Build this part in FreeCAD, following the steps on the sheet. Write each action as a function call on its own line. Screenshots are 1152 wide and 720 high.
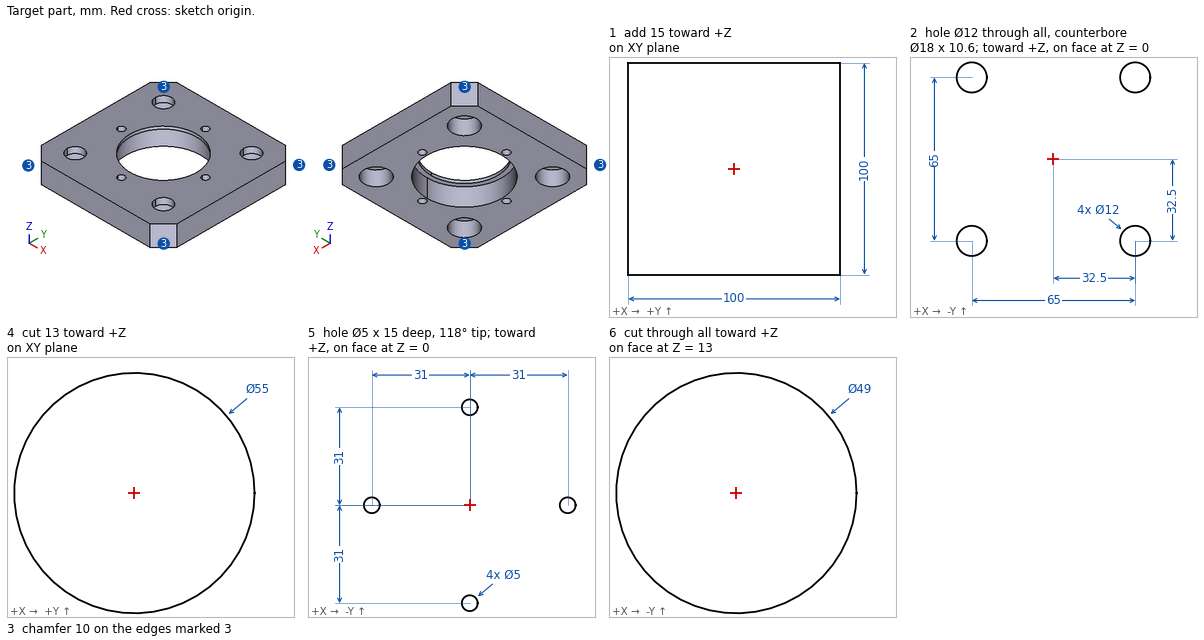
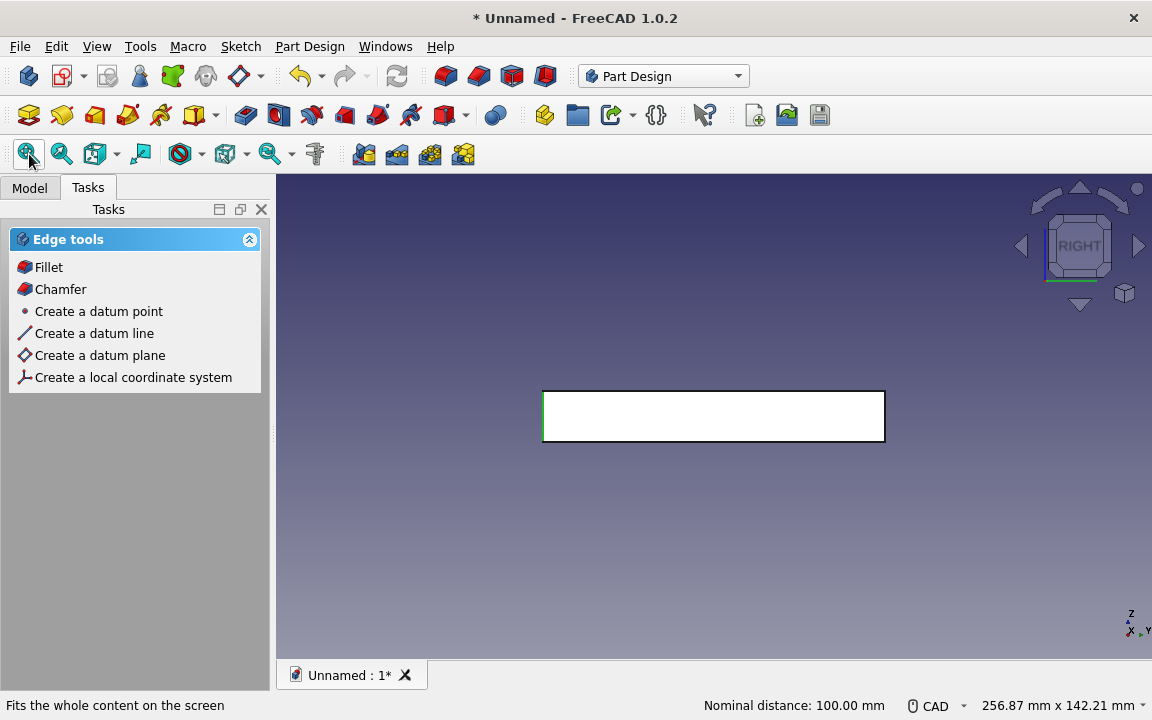
click(885, 415, ctrl)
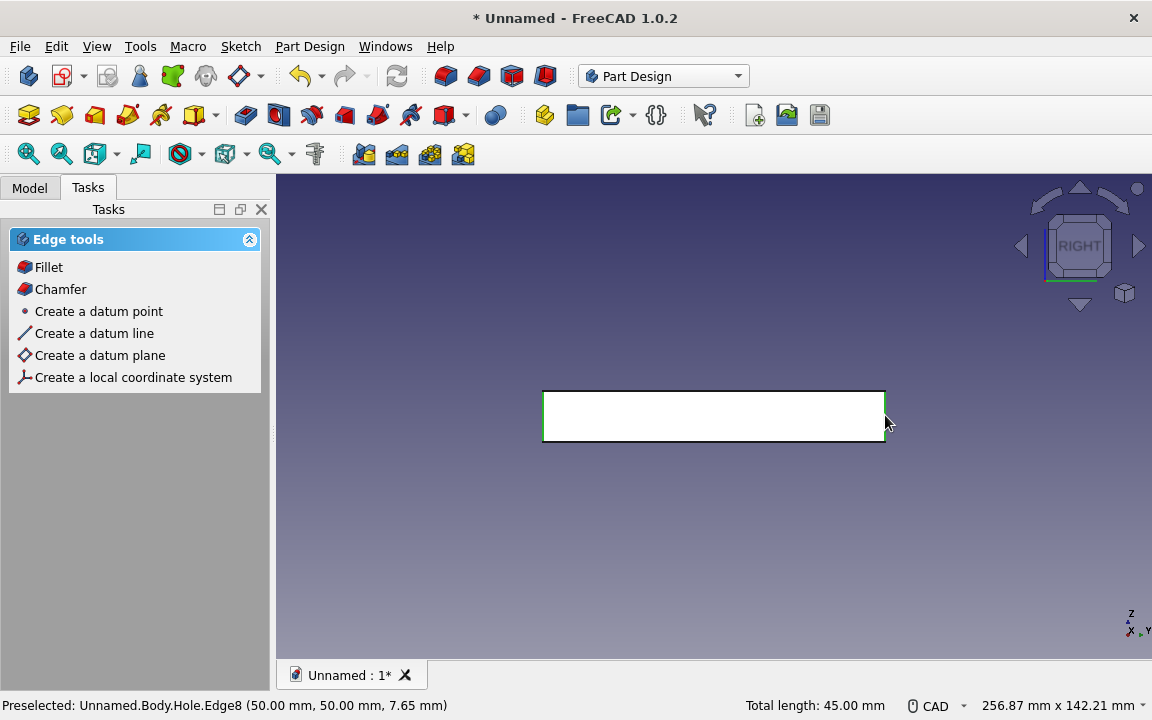
key(5)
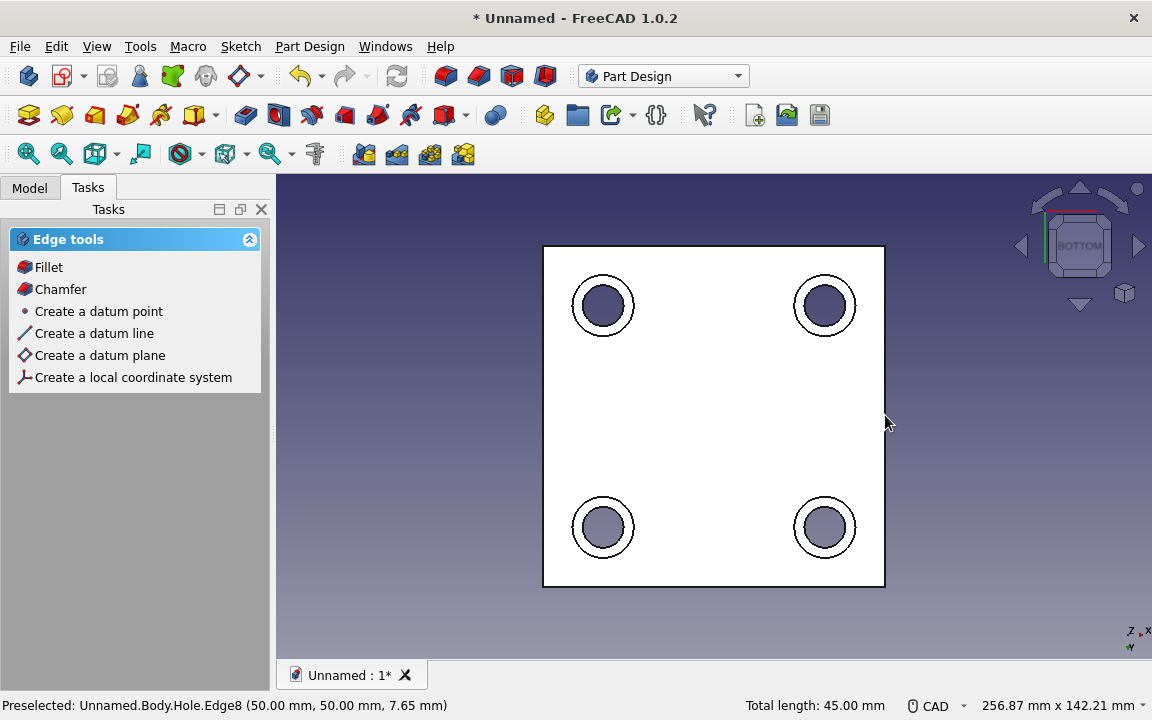
key(4)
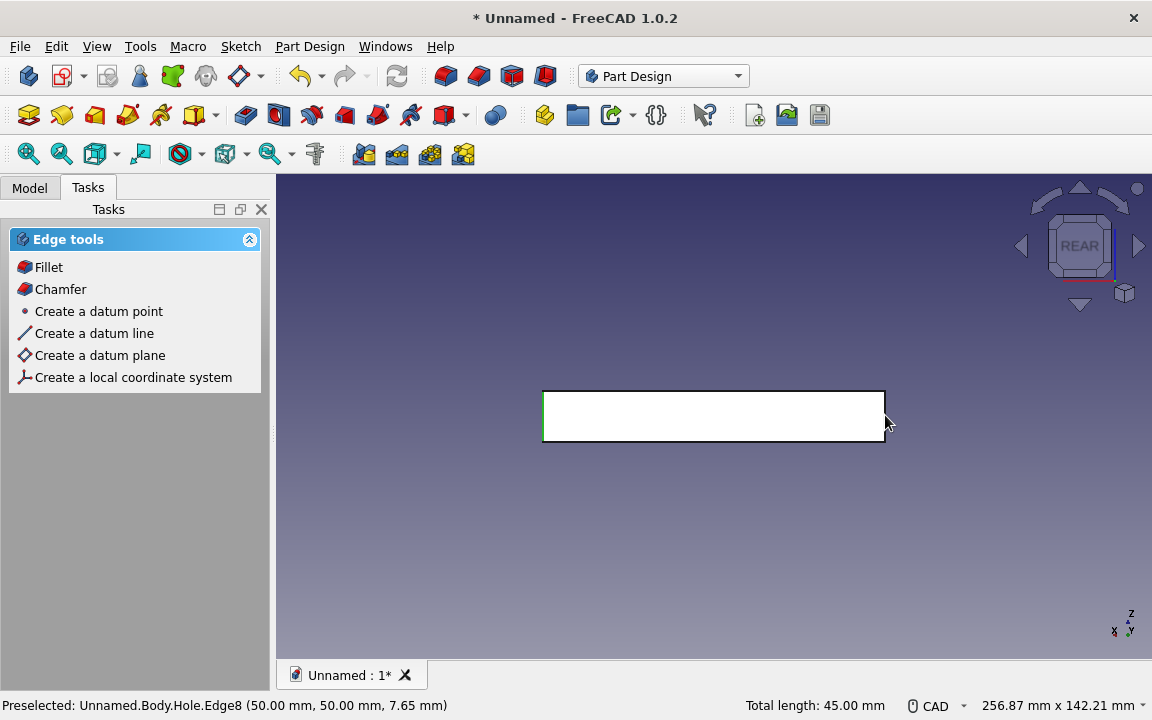
click(29, 154)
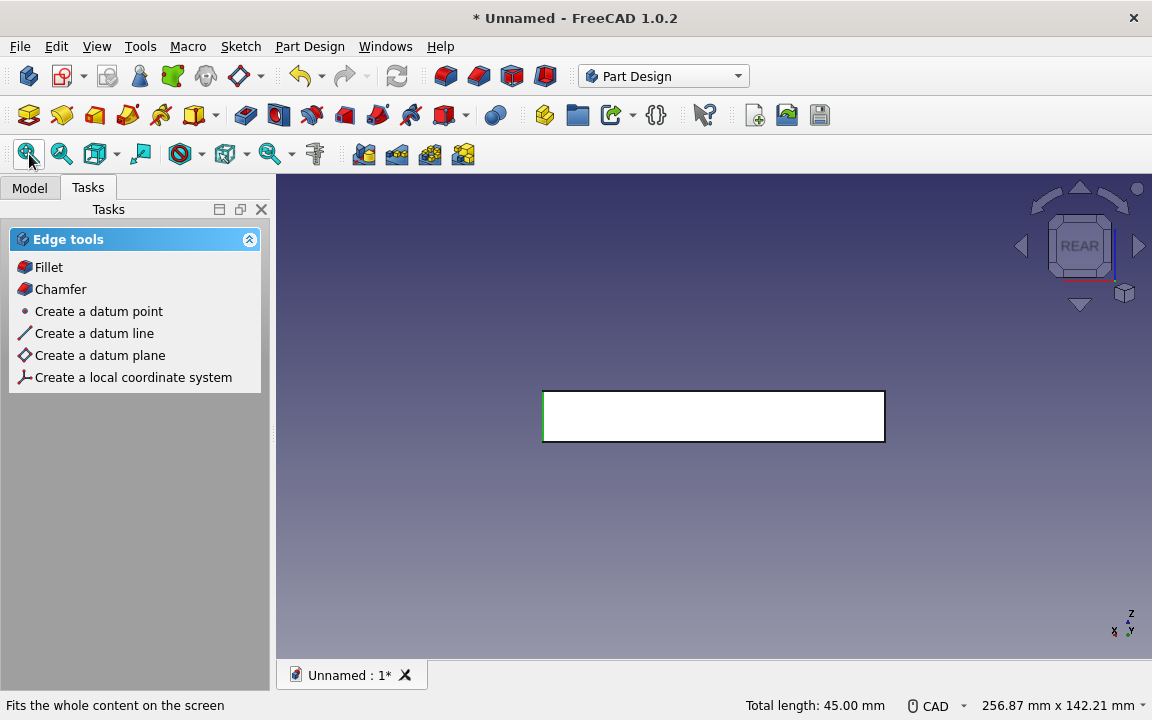
click(885, 416, ctrl)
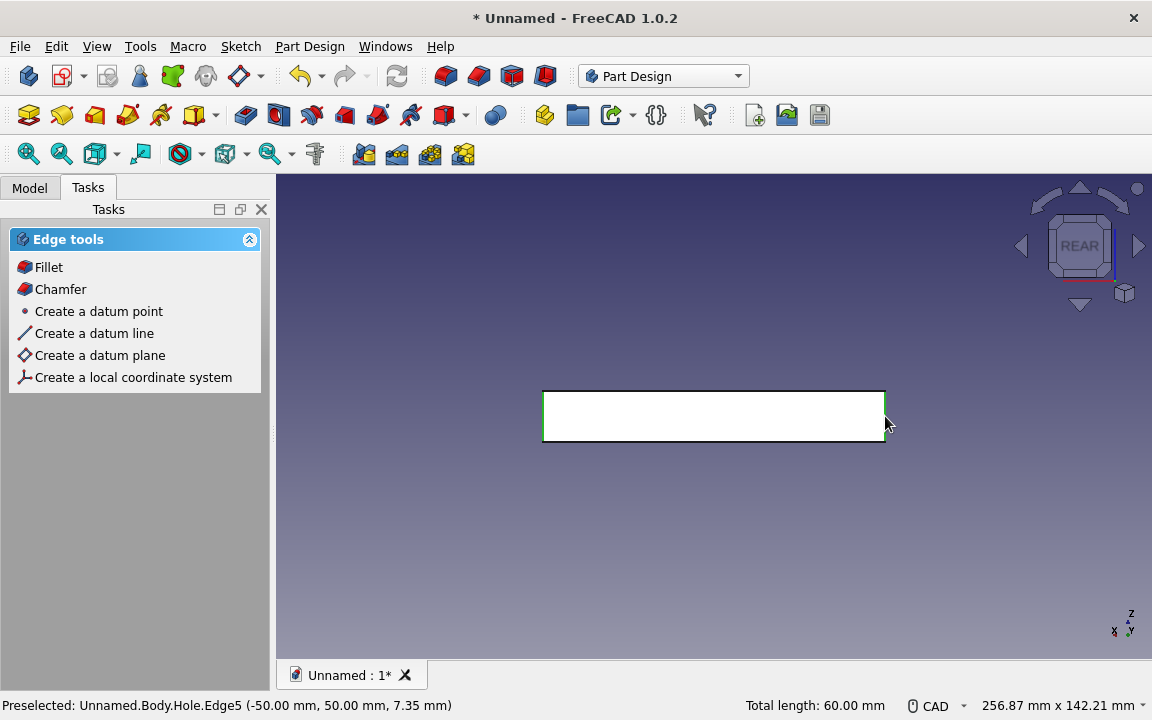
click(479, 76)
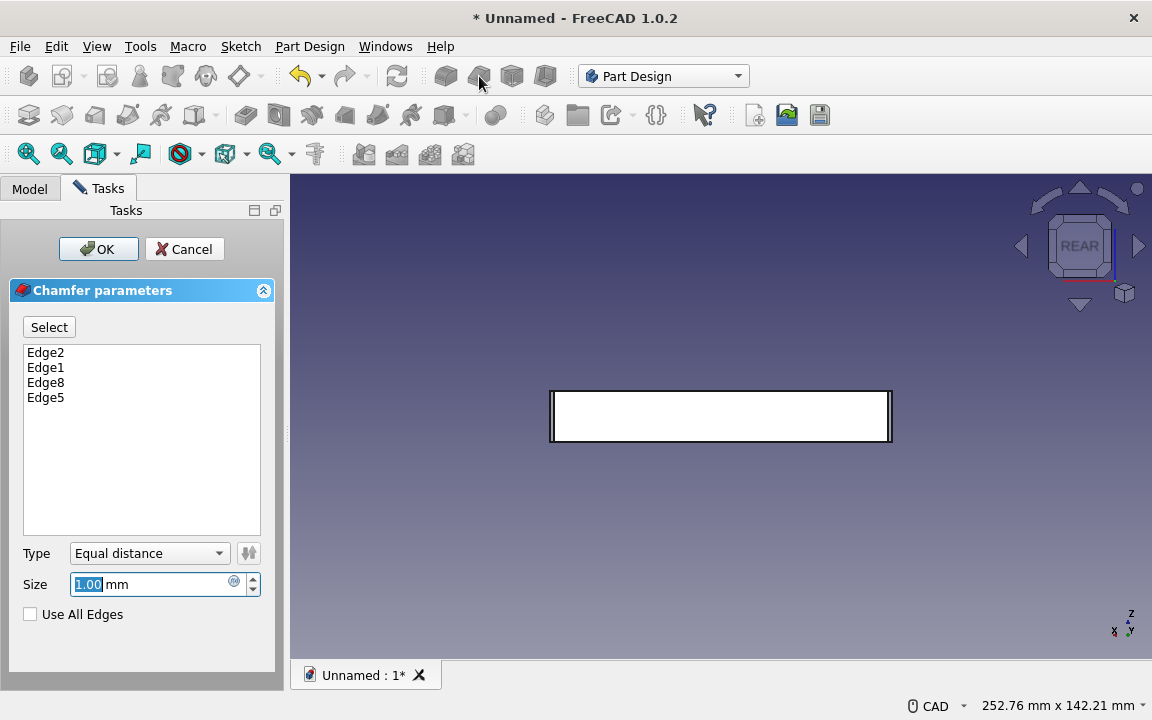
text(10)
key(Tab)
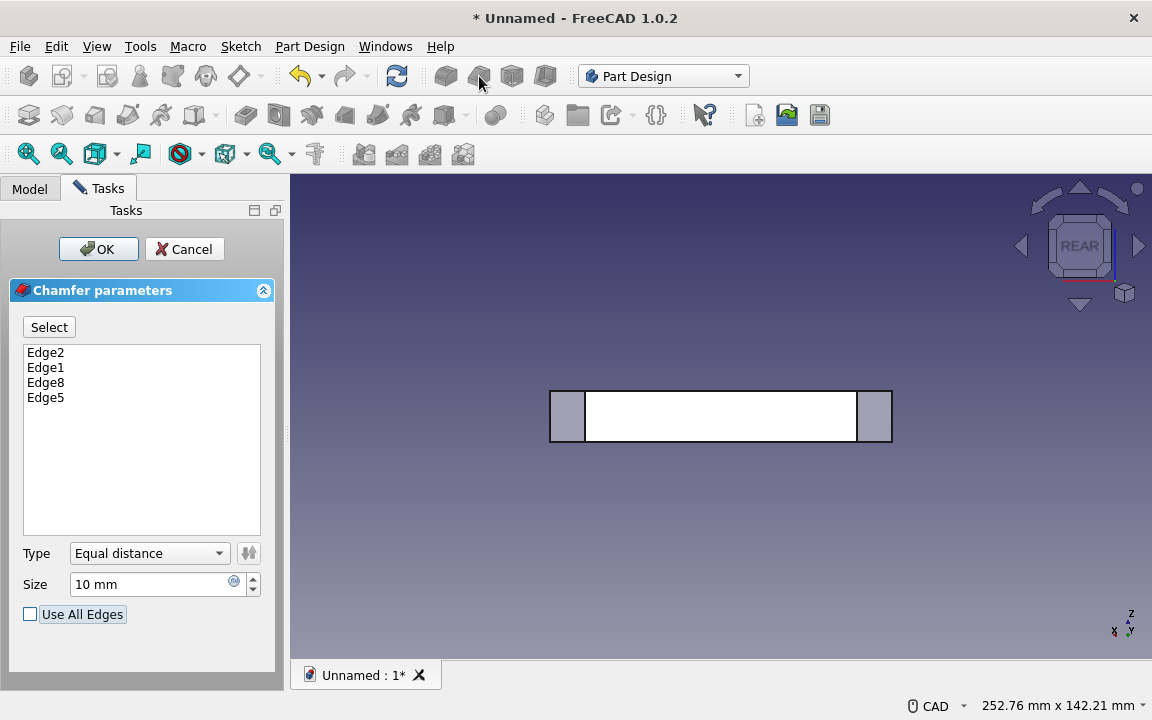
click(99, 249)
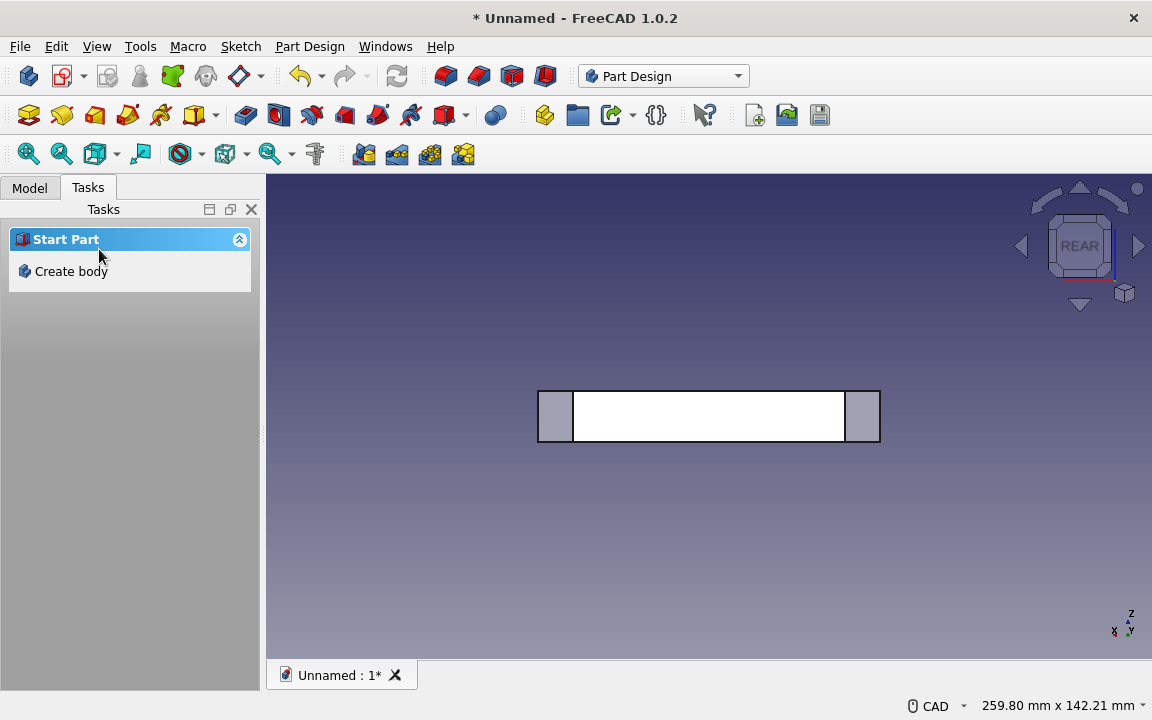
click(29, 154)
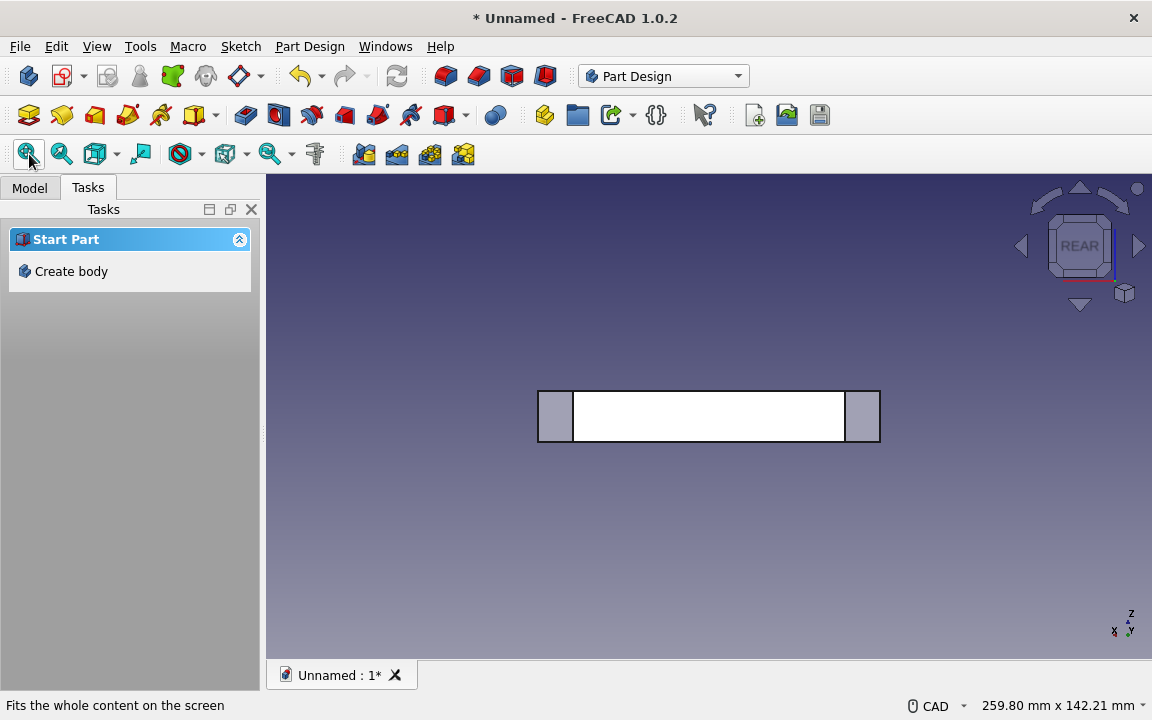
click(62, 76)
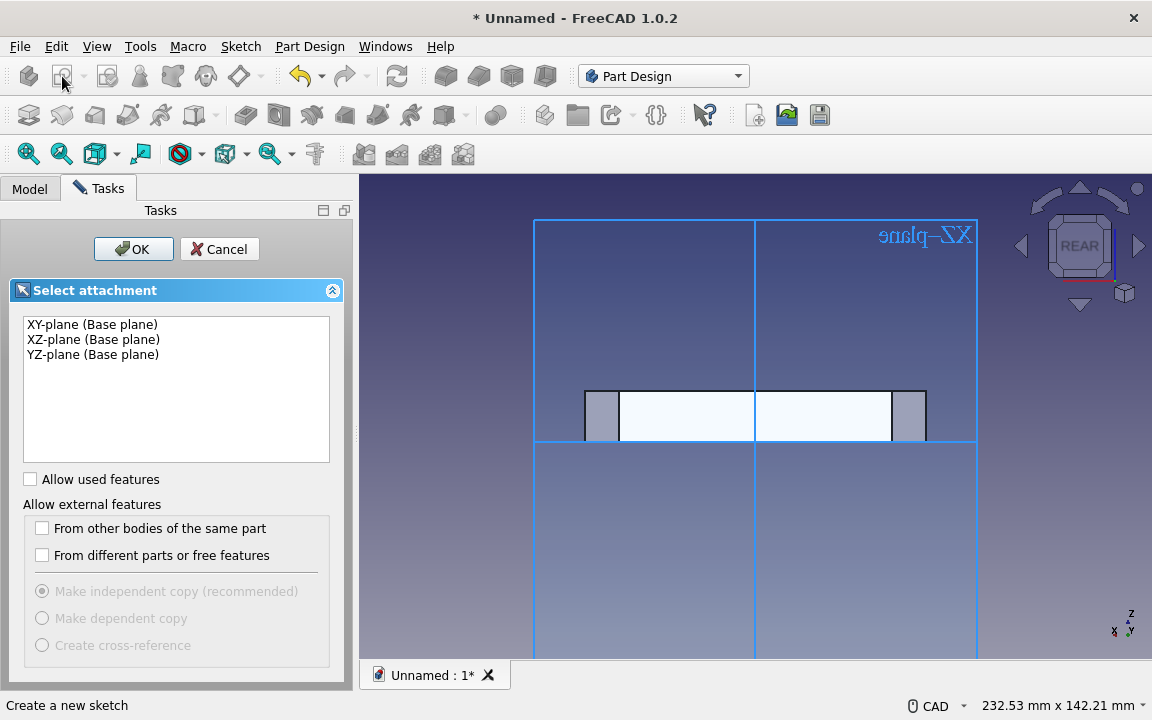
click(84, 324)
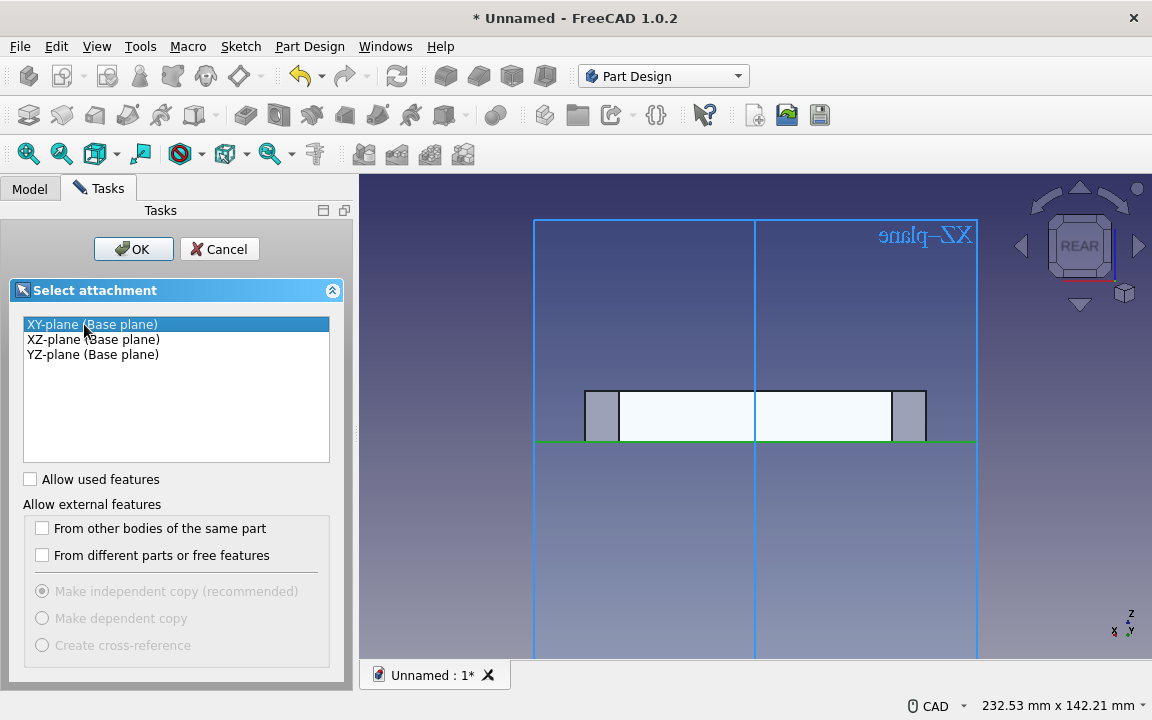
click(134, 249)